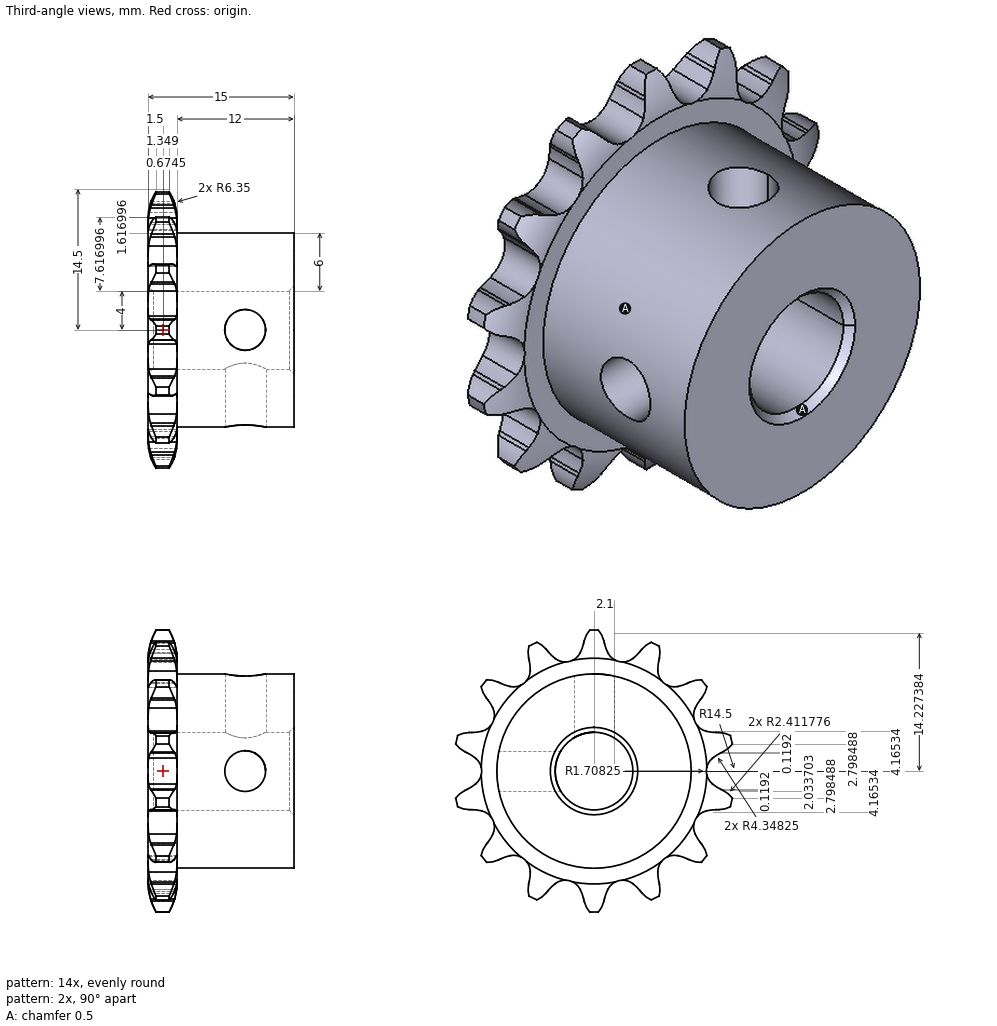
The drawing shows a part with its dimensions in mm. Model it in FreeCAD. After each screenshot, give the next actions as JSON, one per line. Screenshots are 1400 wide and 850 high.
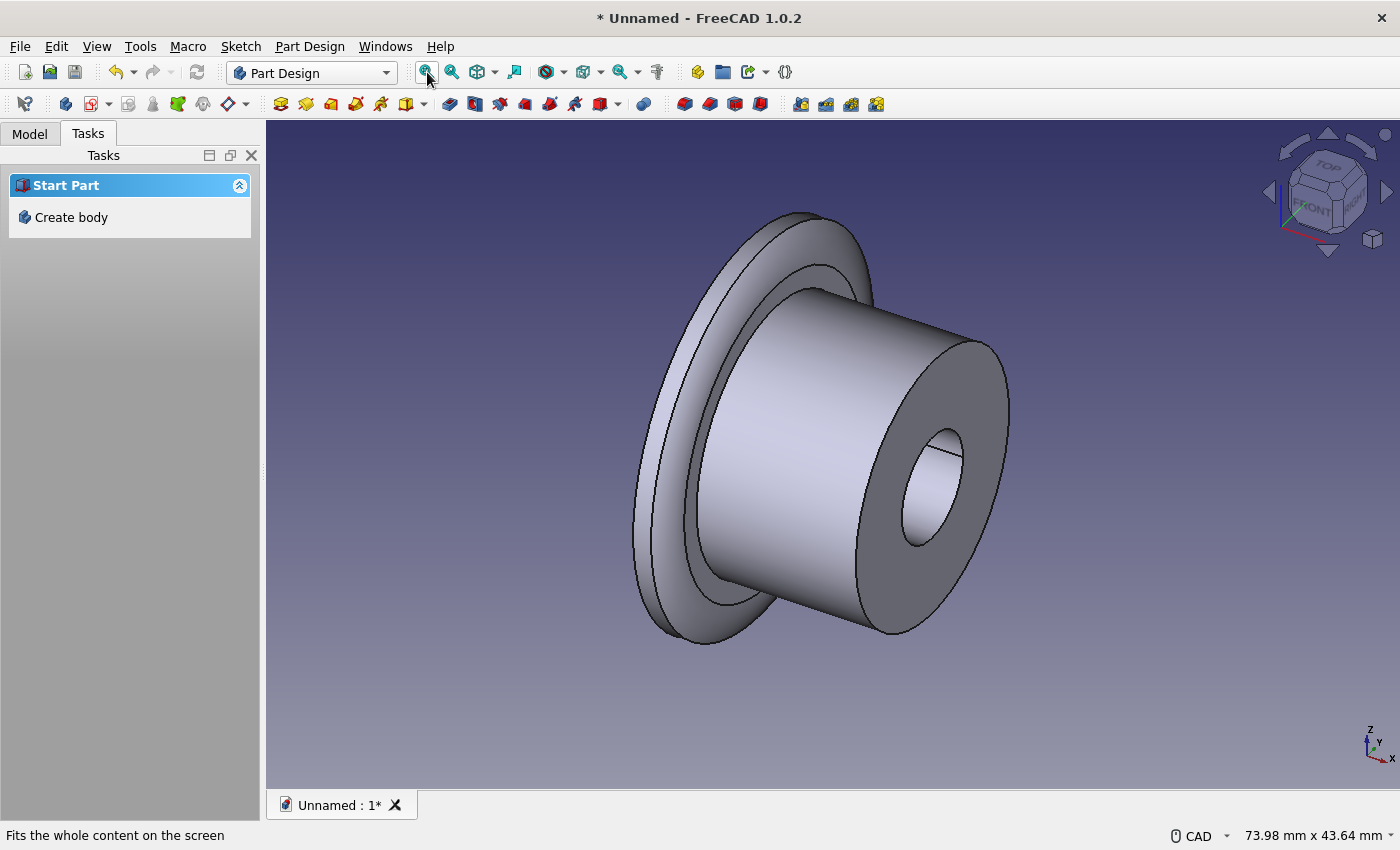
{"action": "left_click", "coordinate": [90, 104]}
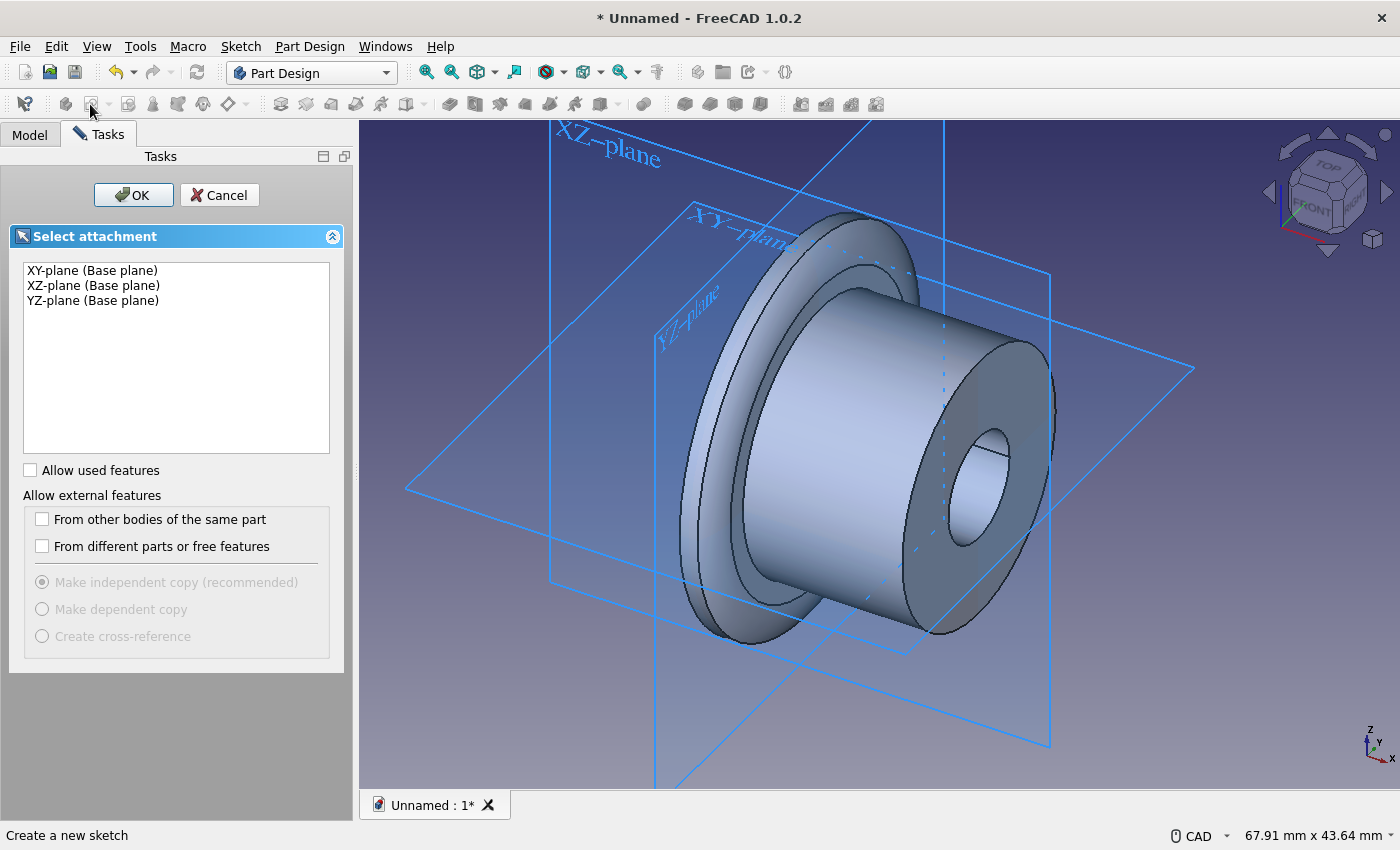
{"action": "left_click", "coordinate": [84, 300]}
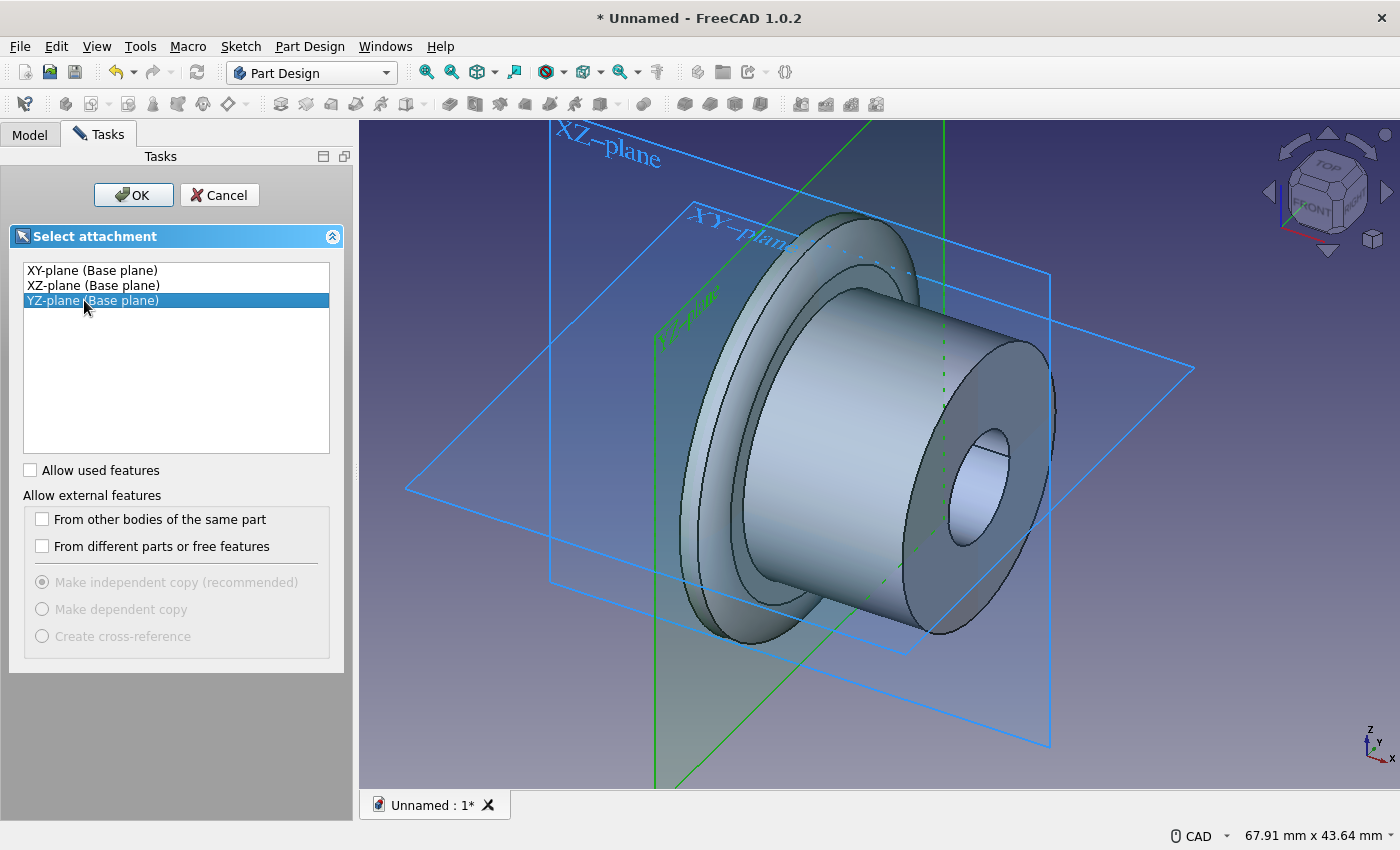
{"action": "left_click", "coordinate": [134, 195]}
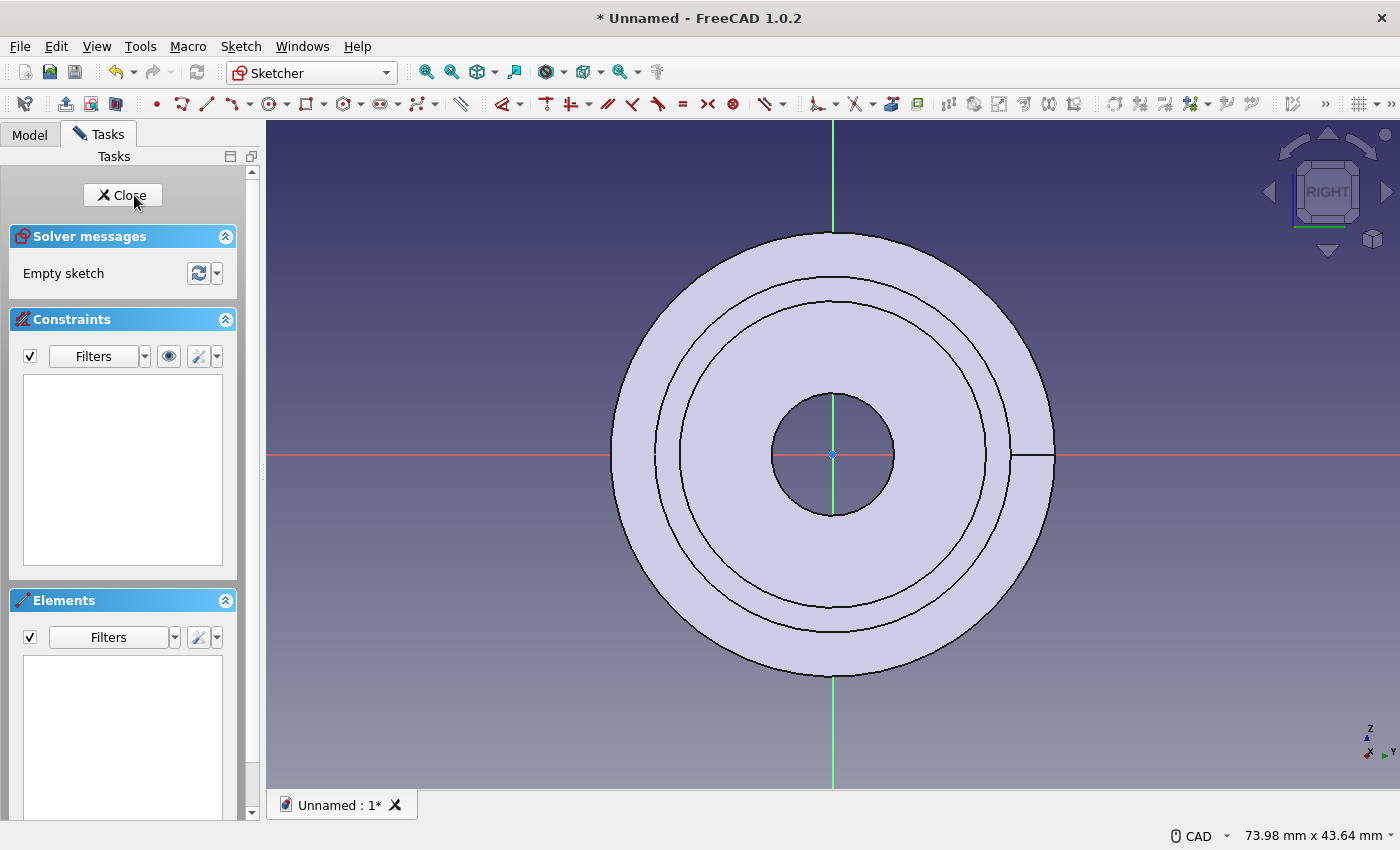
{"action": "left_click", "coordinate": [116, 104]}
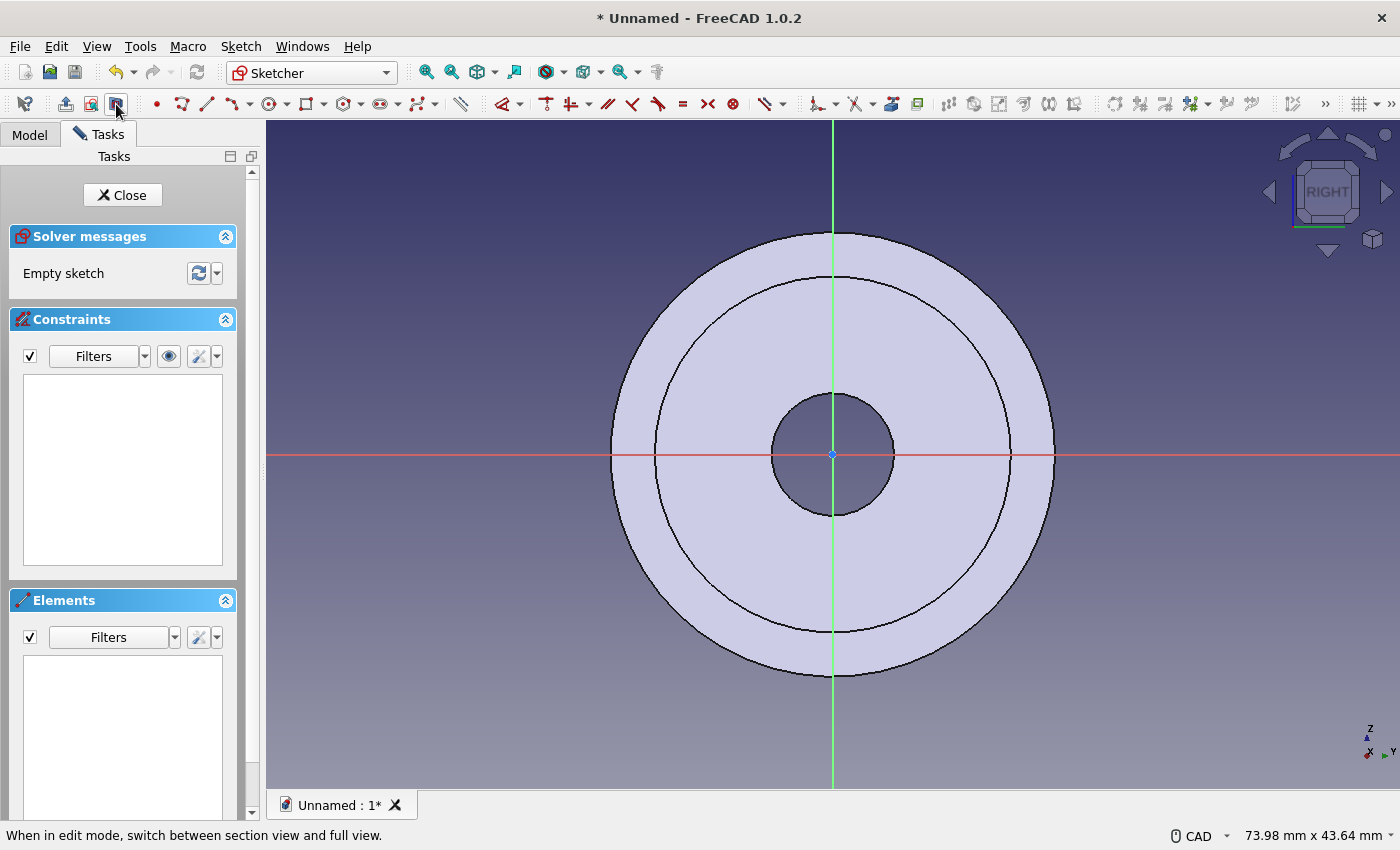
{"action": "scroll", "coordinate": [1100, 454], "scroll_direction": "up", "scroll_amount": 8}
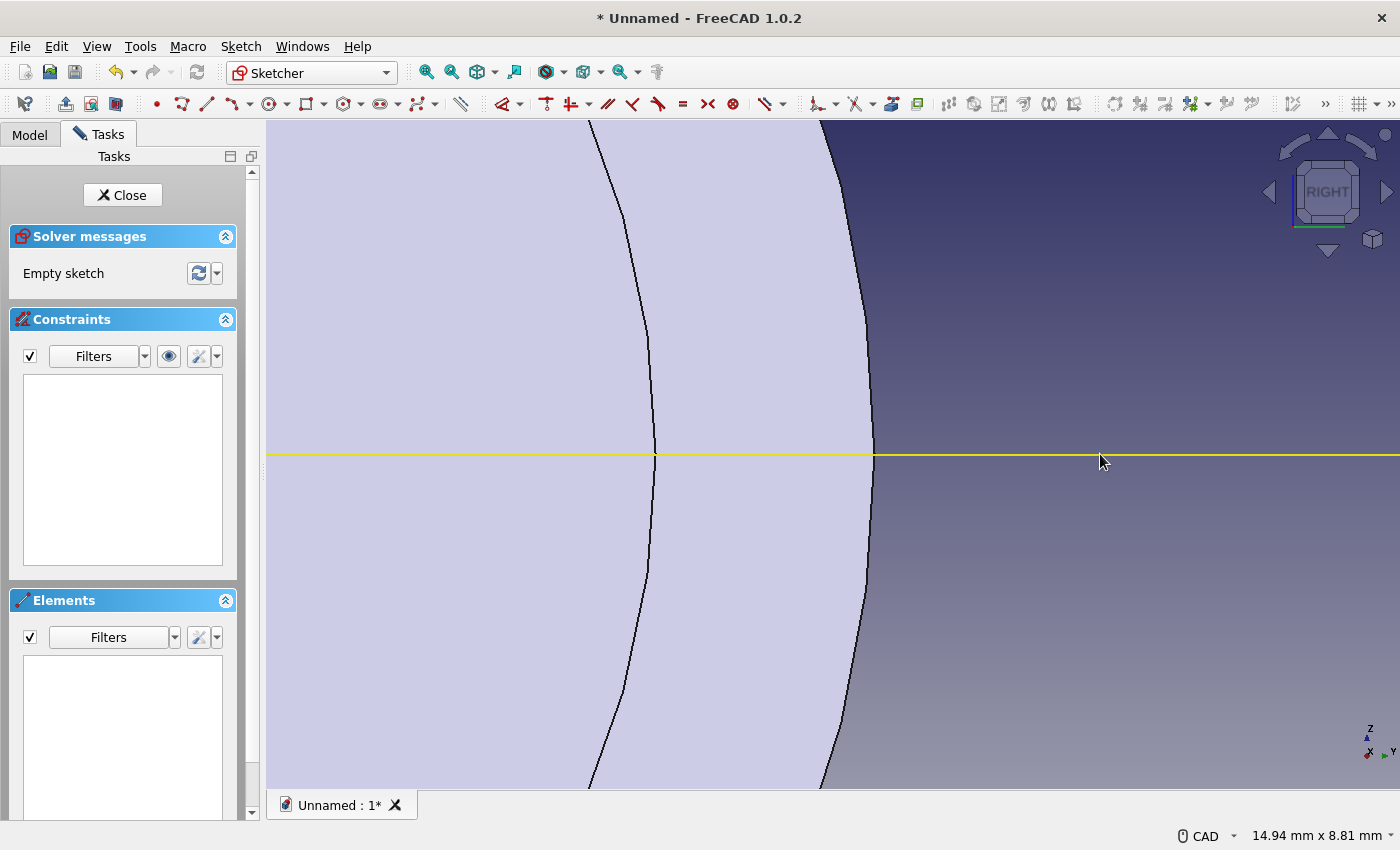
{"action": "left_click", "coordinate": [207, 104]}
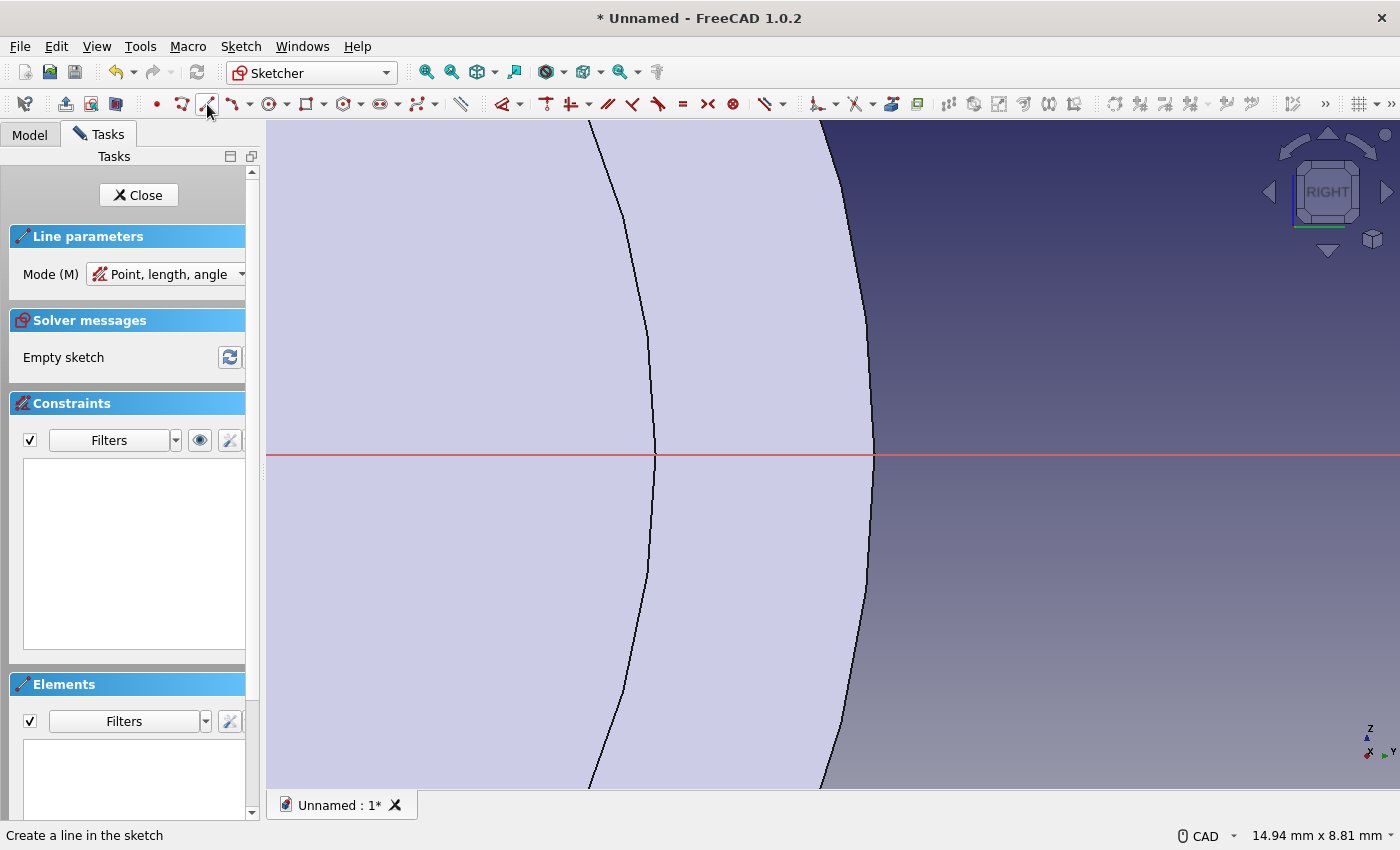
{"action": "left_click", "coordinate": [764, 597]}
{"action": "left_click", "coordinate": [783, 606]}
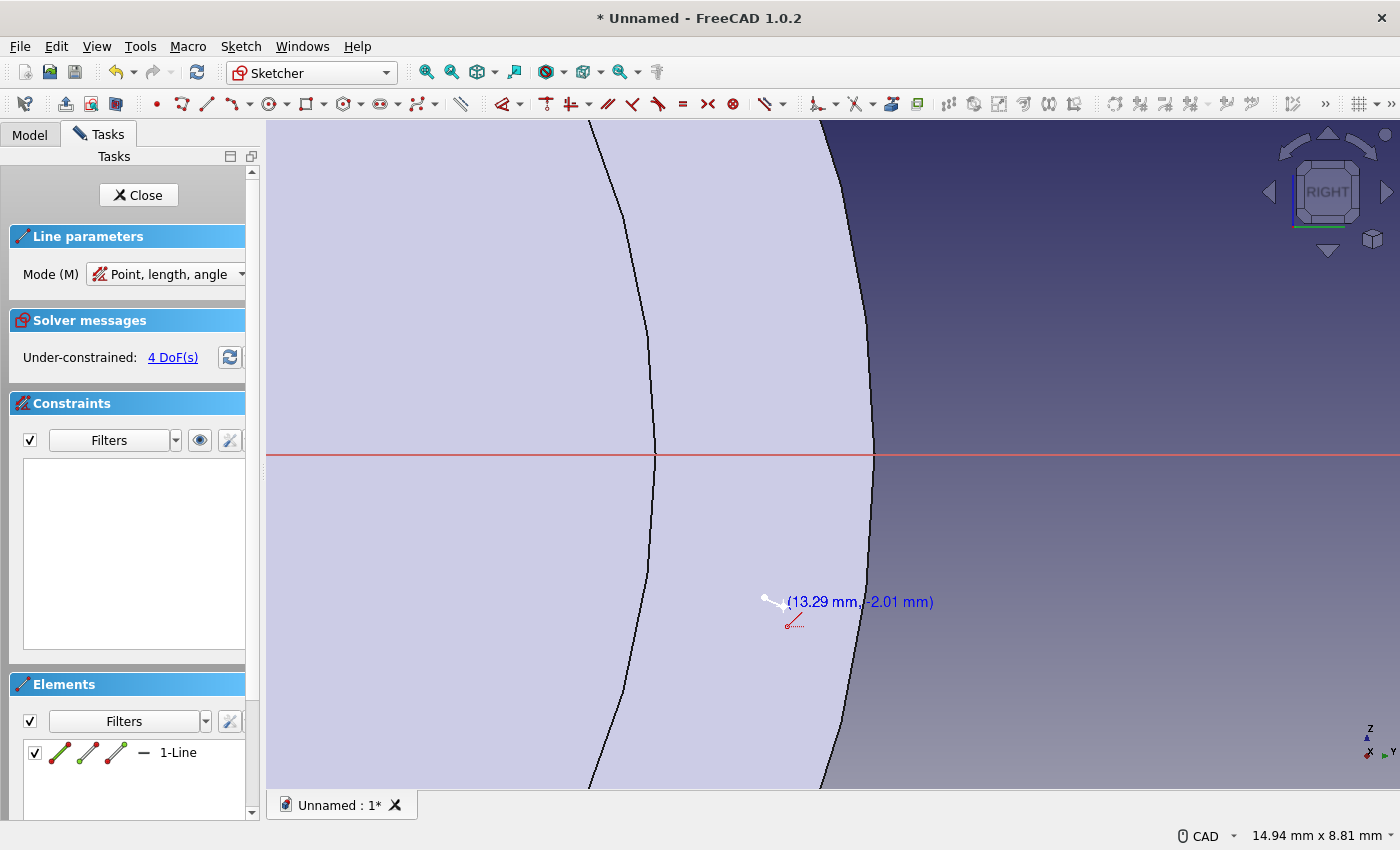
{"action": "left_click", "coordinate": [783, 303]}
{"action": "left_click", "coordinate": [764, 312]}